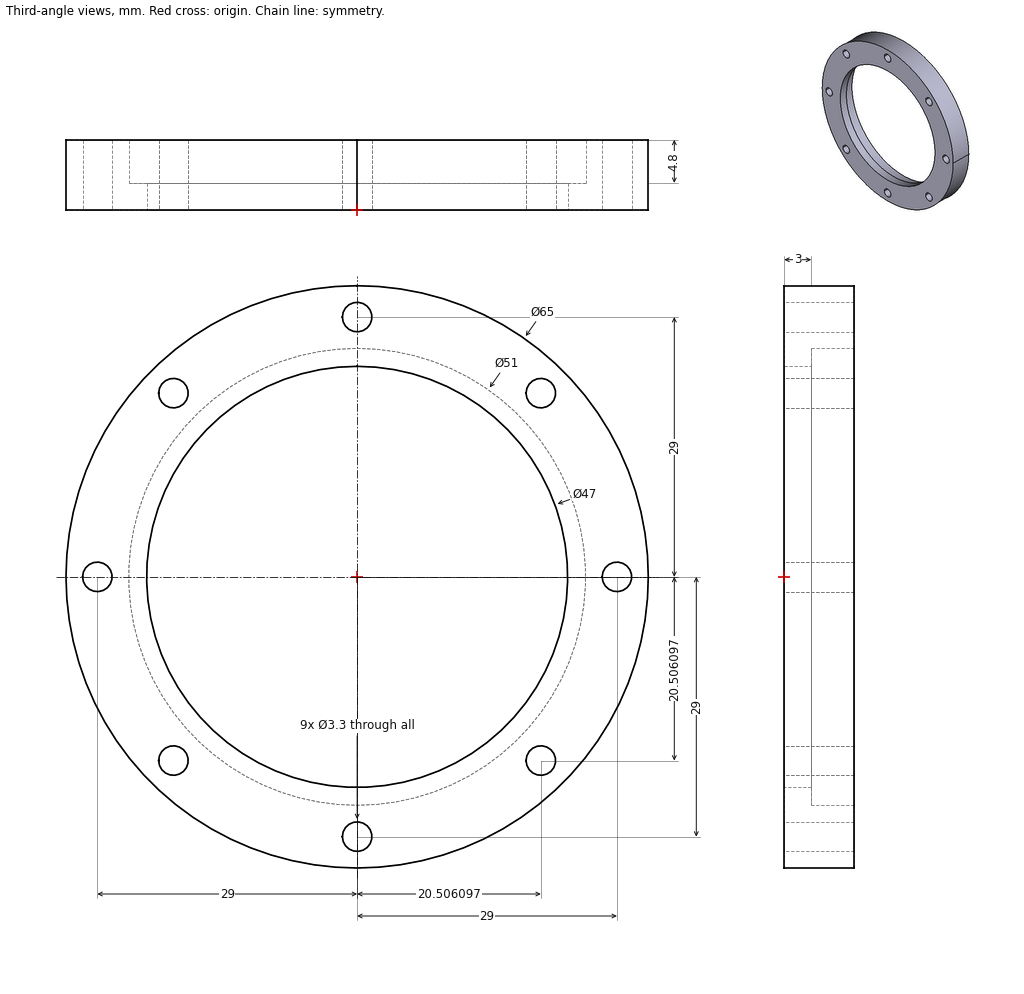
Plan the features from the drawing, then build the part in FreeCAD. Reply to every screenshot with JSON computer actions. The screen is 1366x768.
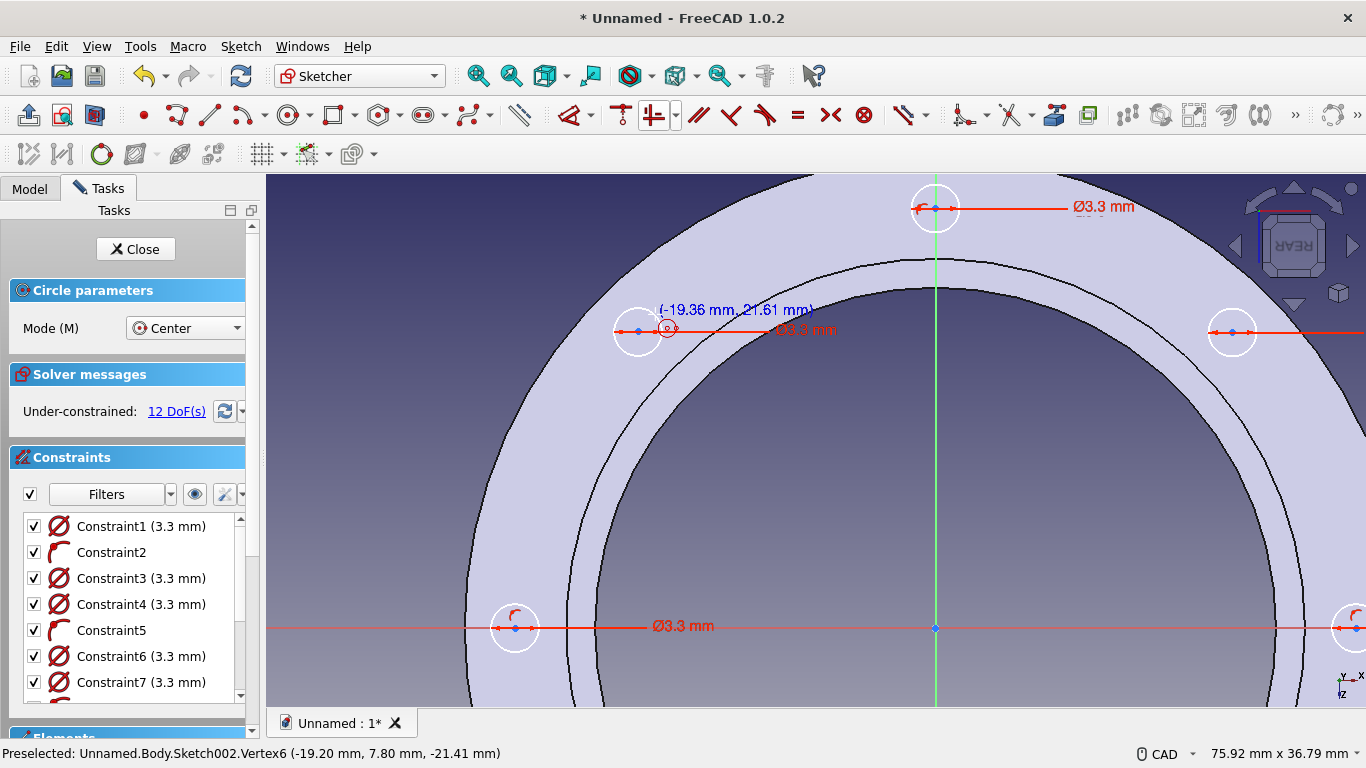
{"action": "left_click", "coordinate": [936, 628]}
{"action": "mouse_move", "coordinate": [952, 611]}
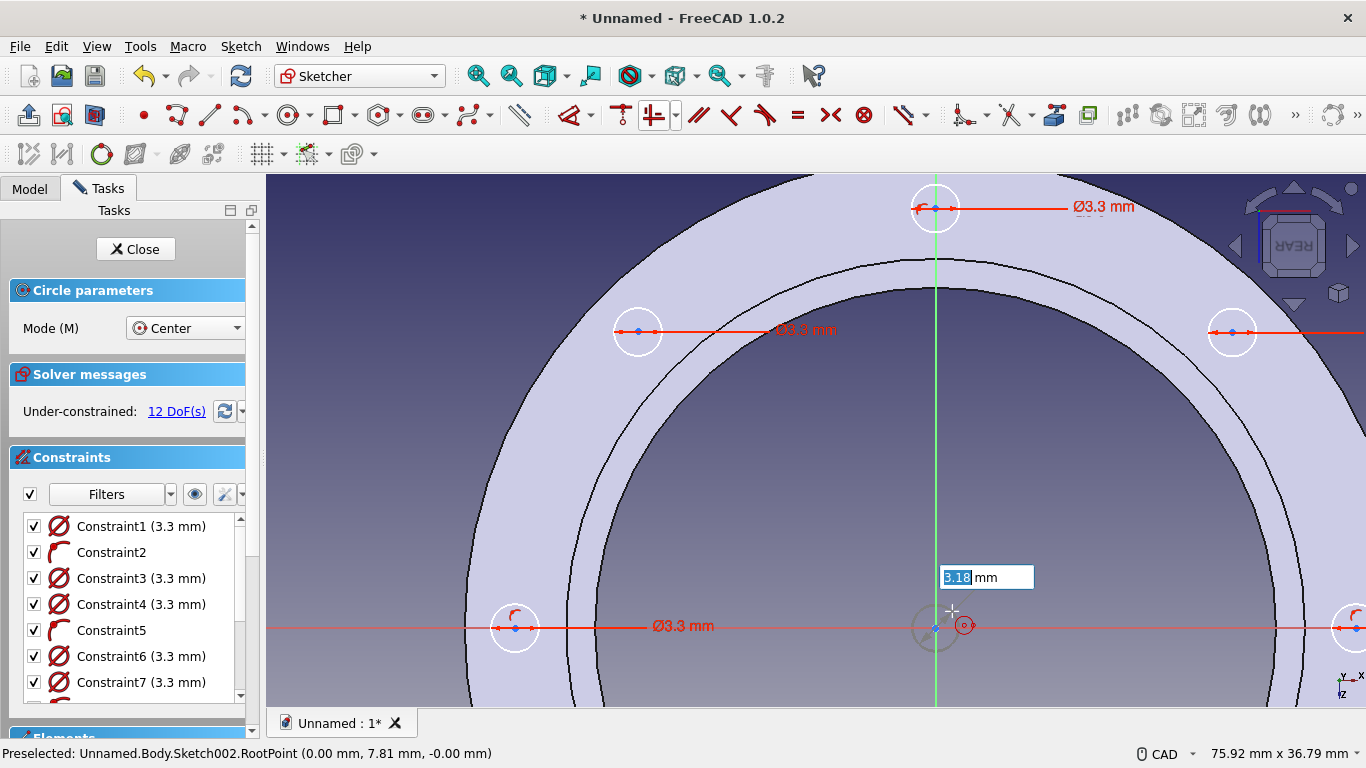
{"action": "type", "text": "3.3"}
{"action": "key", "text": "Return"}
{"action": "key", "text": "Escape"}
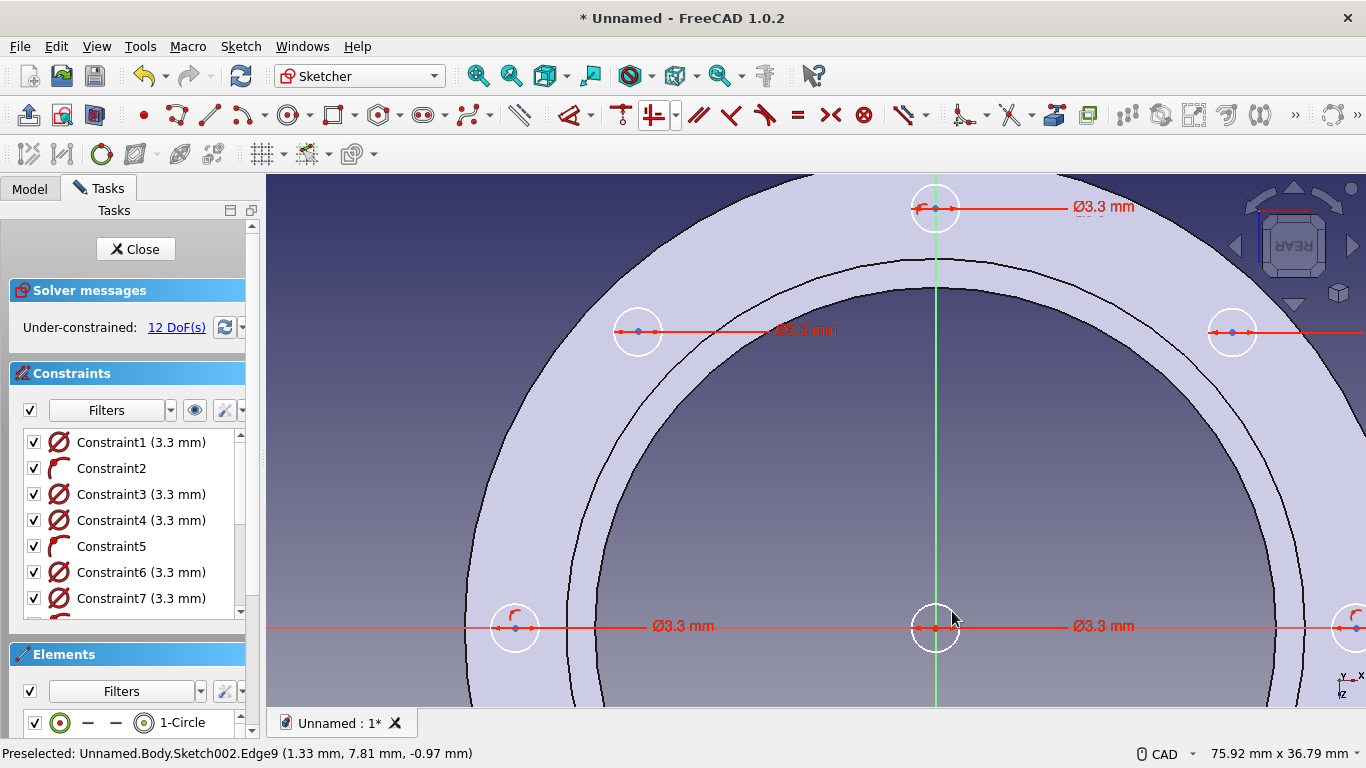
{"action": "scroll", "coordinate": [638, 331], "scroll_direction": "down", "scroll_amount": 5}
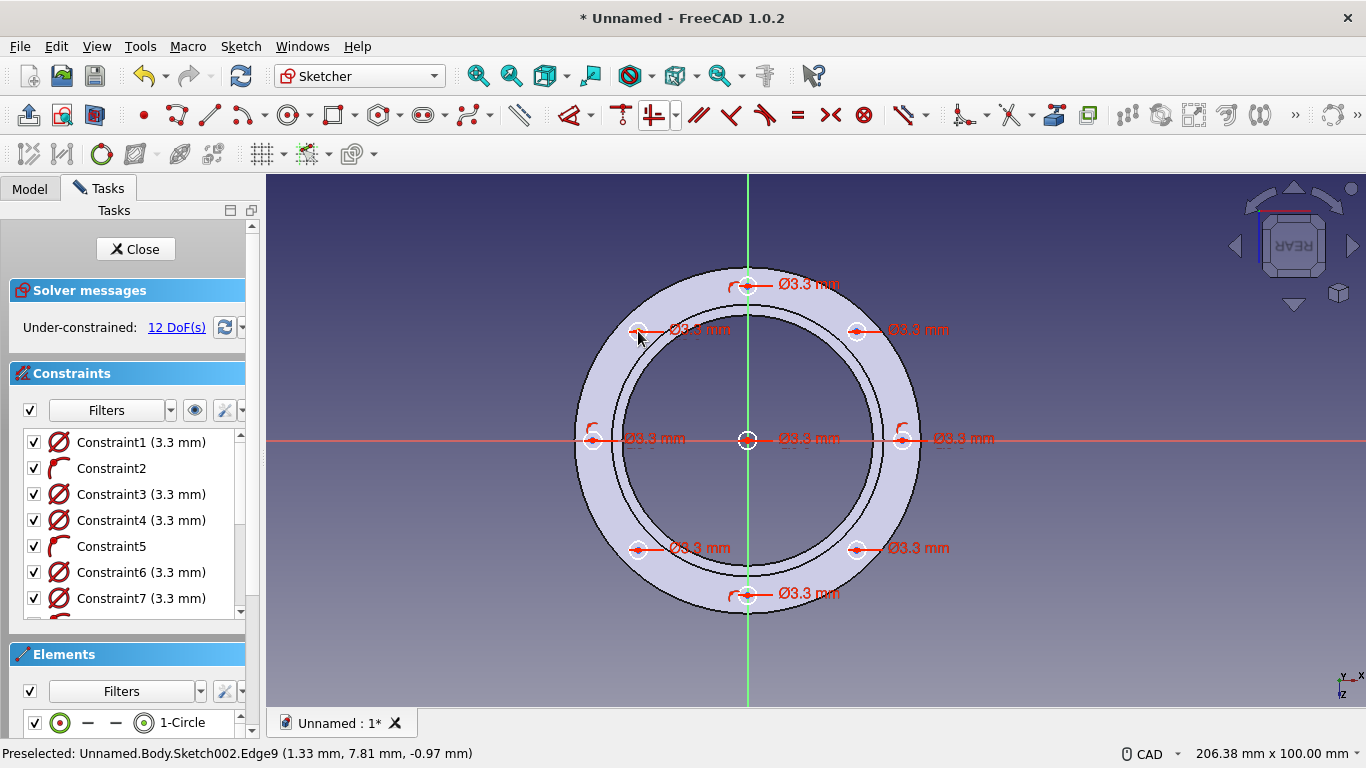
{"action": "left_click", "coordinate": [857, 332]}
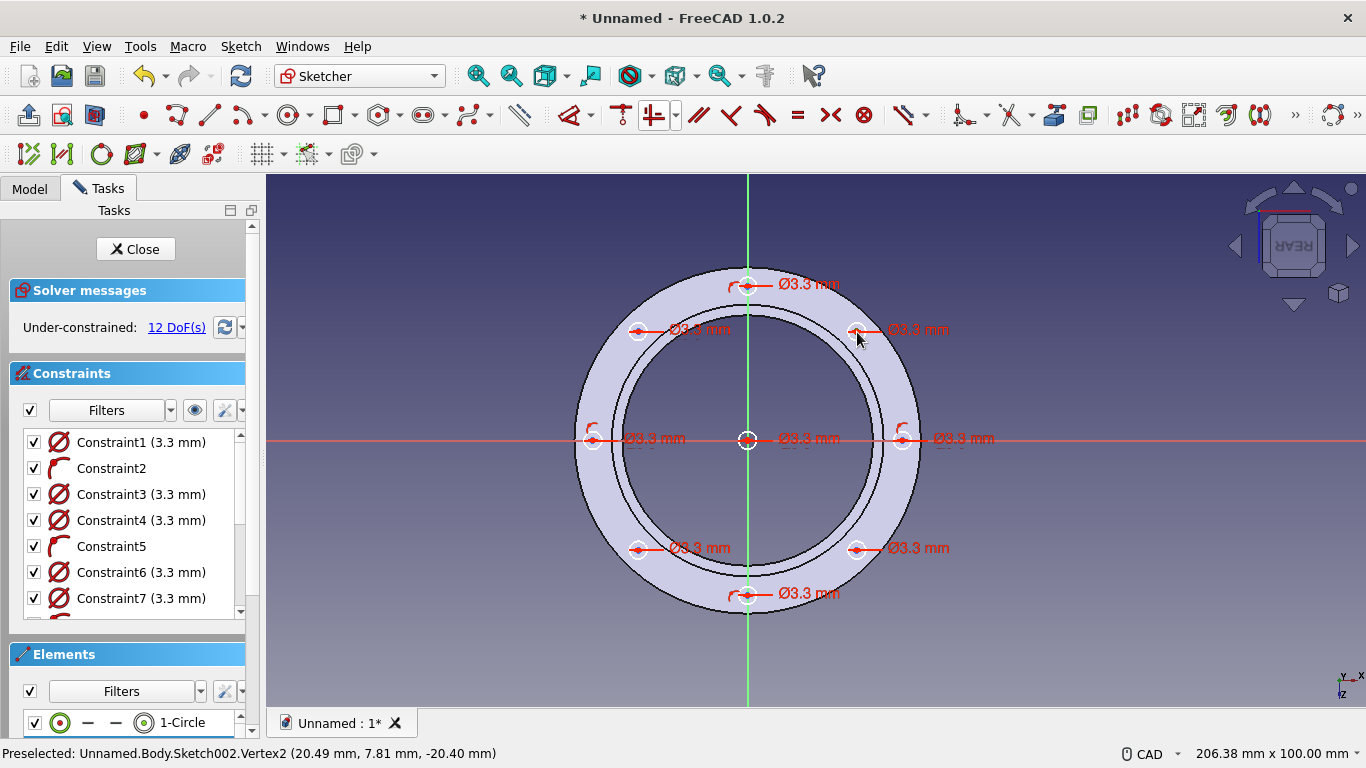
{"action": "left_click", "coordinate": [857, 550]}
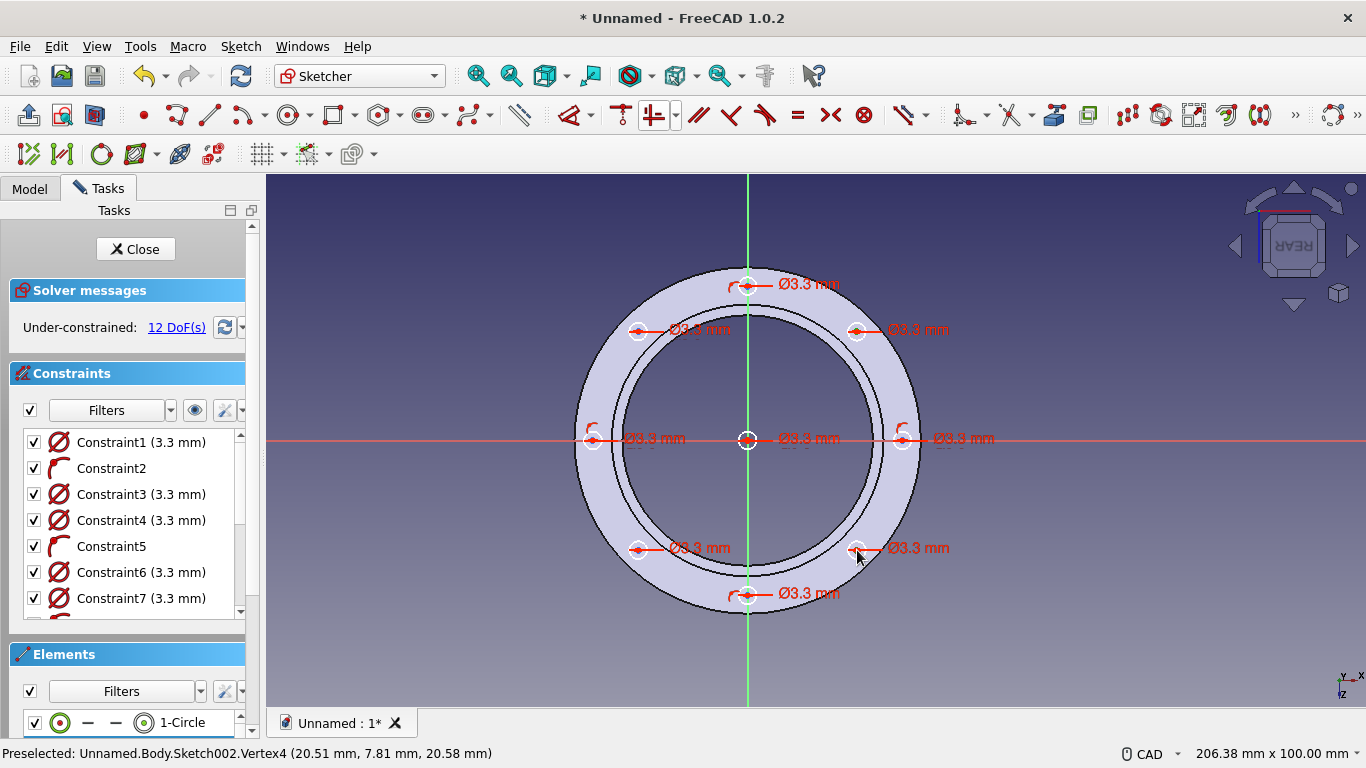
{"action": "left_click", "coordinate": [359, 440]}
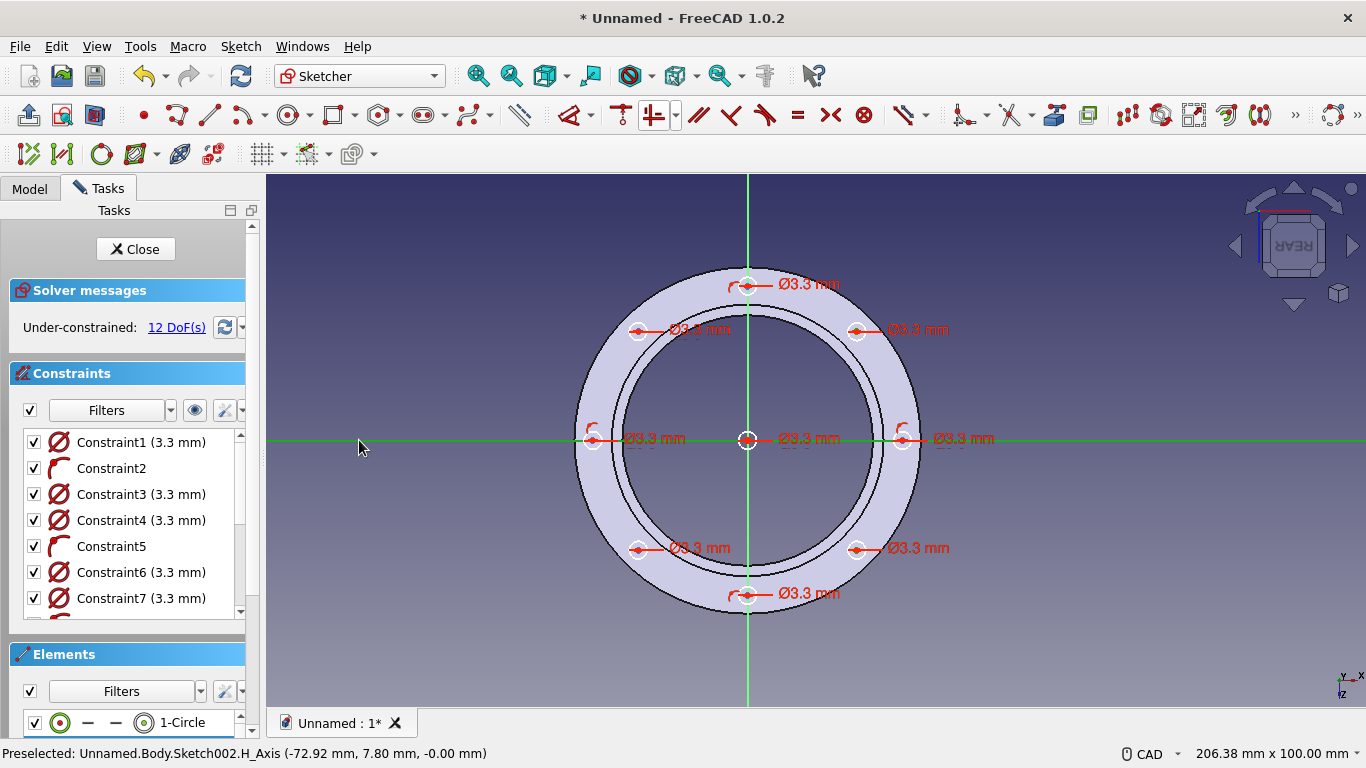
{"action": "left_click", "coordinate": [831, 116]}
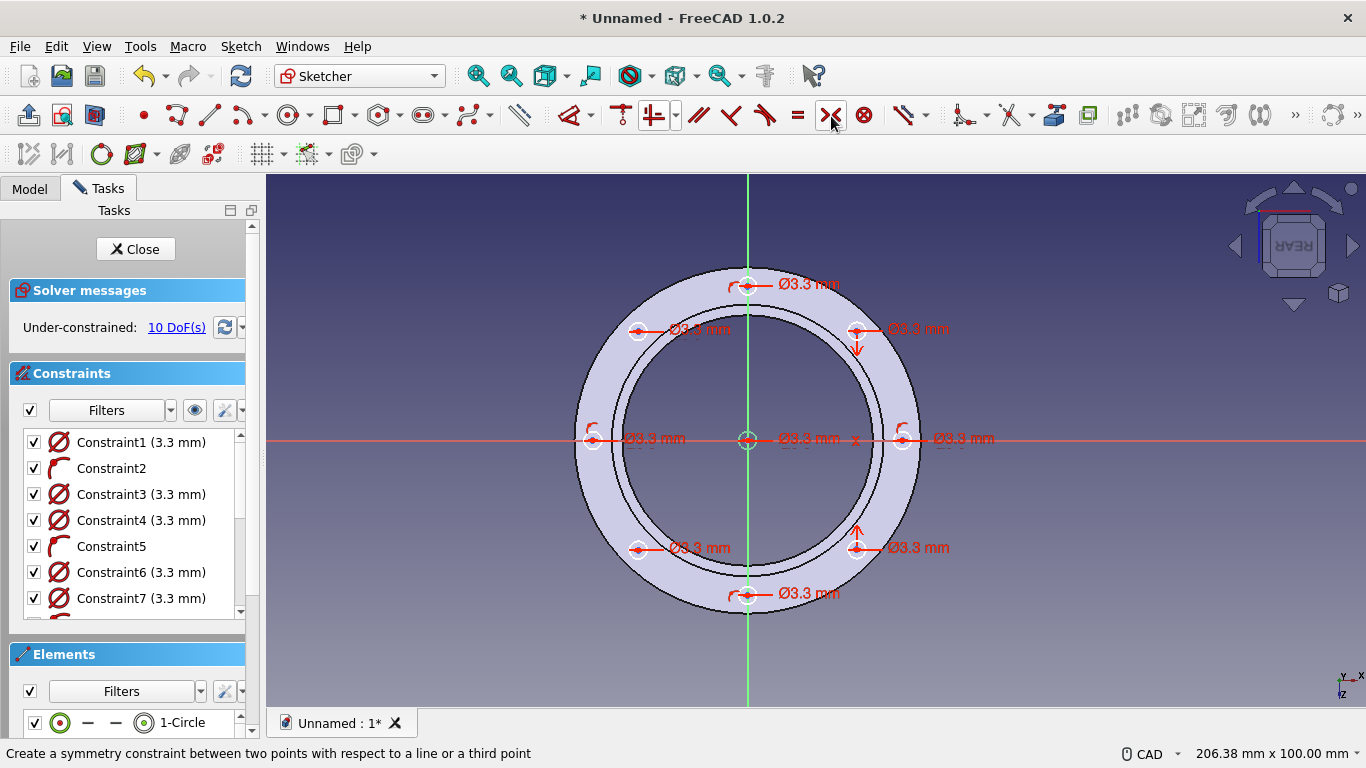
{"action": "left_click", "coordinate": [857, 550]}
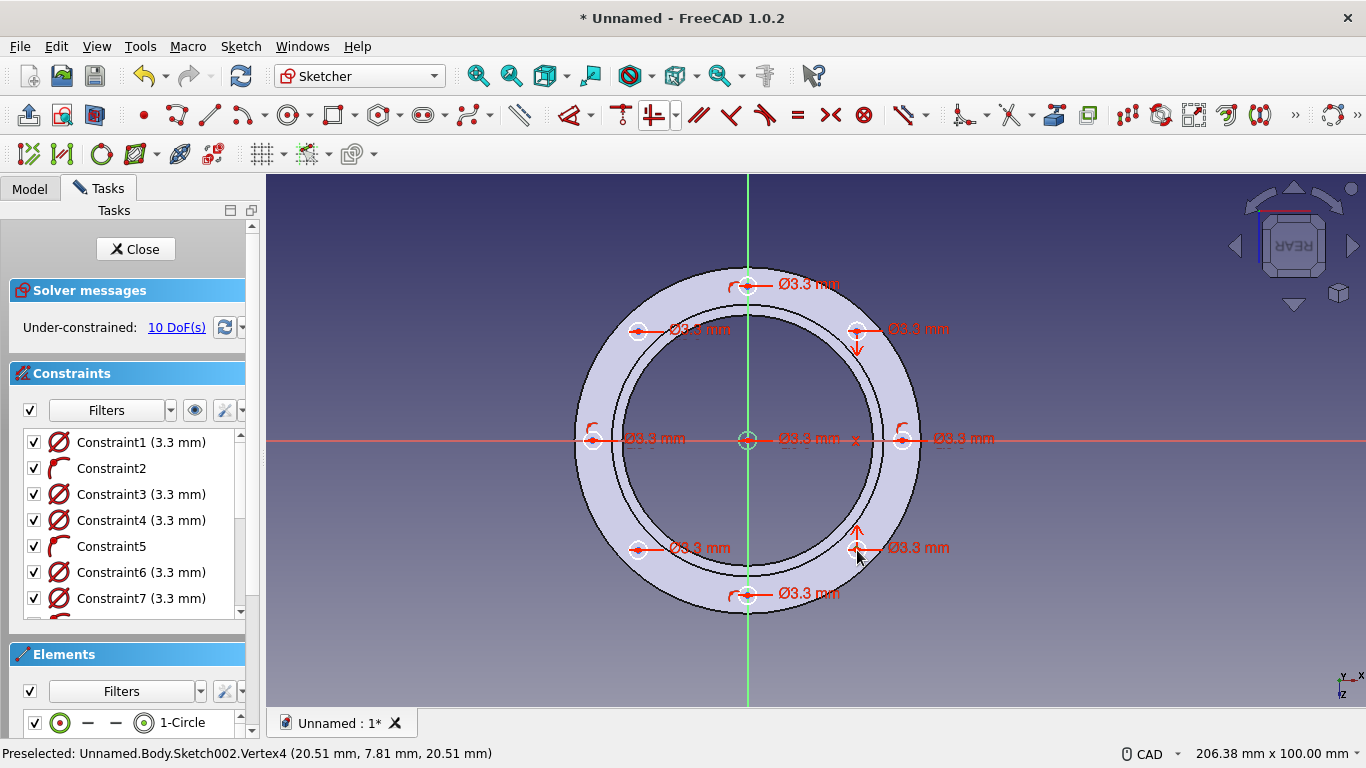
{"action": "left_click", "coordinate": [638, 550]}